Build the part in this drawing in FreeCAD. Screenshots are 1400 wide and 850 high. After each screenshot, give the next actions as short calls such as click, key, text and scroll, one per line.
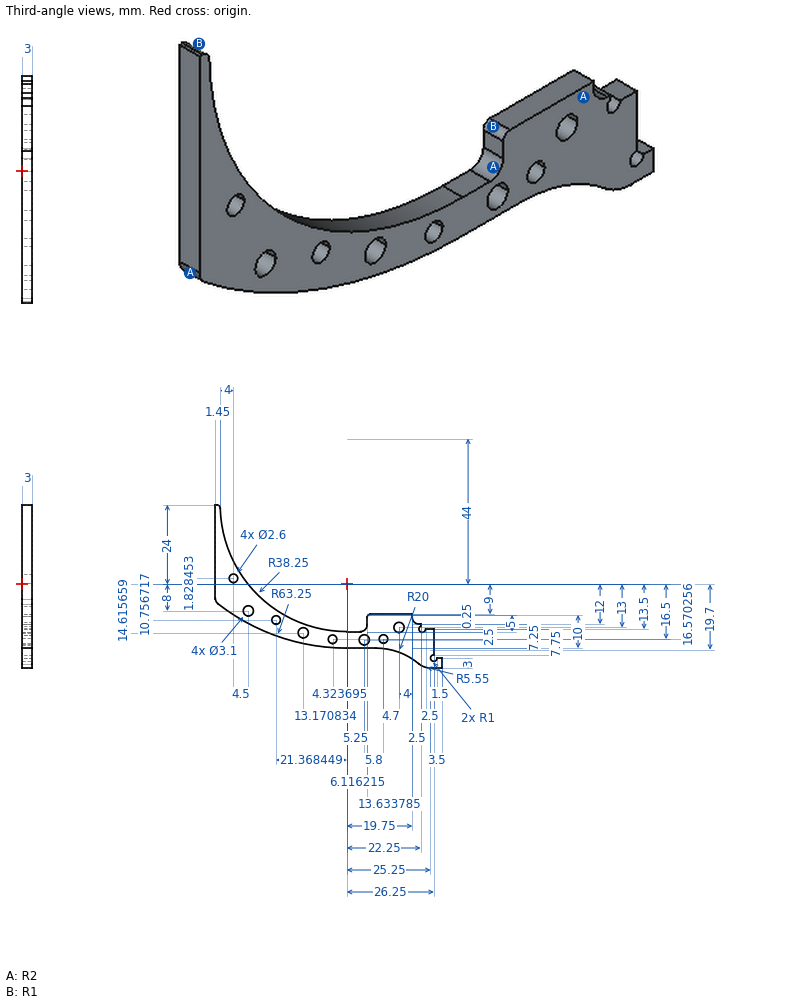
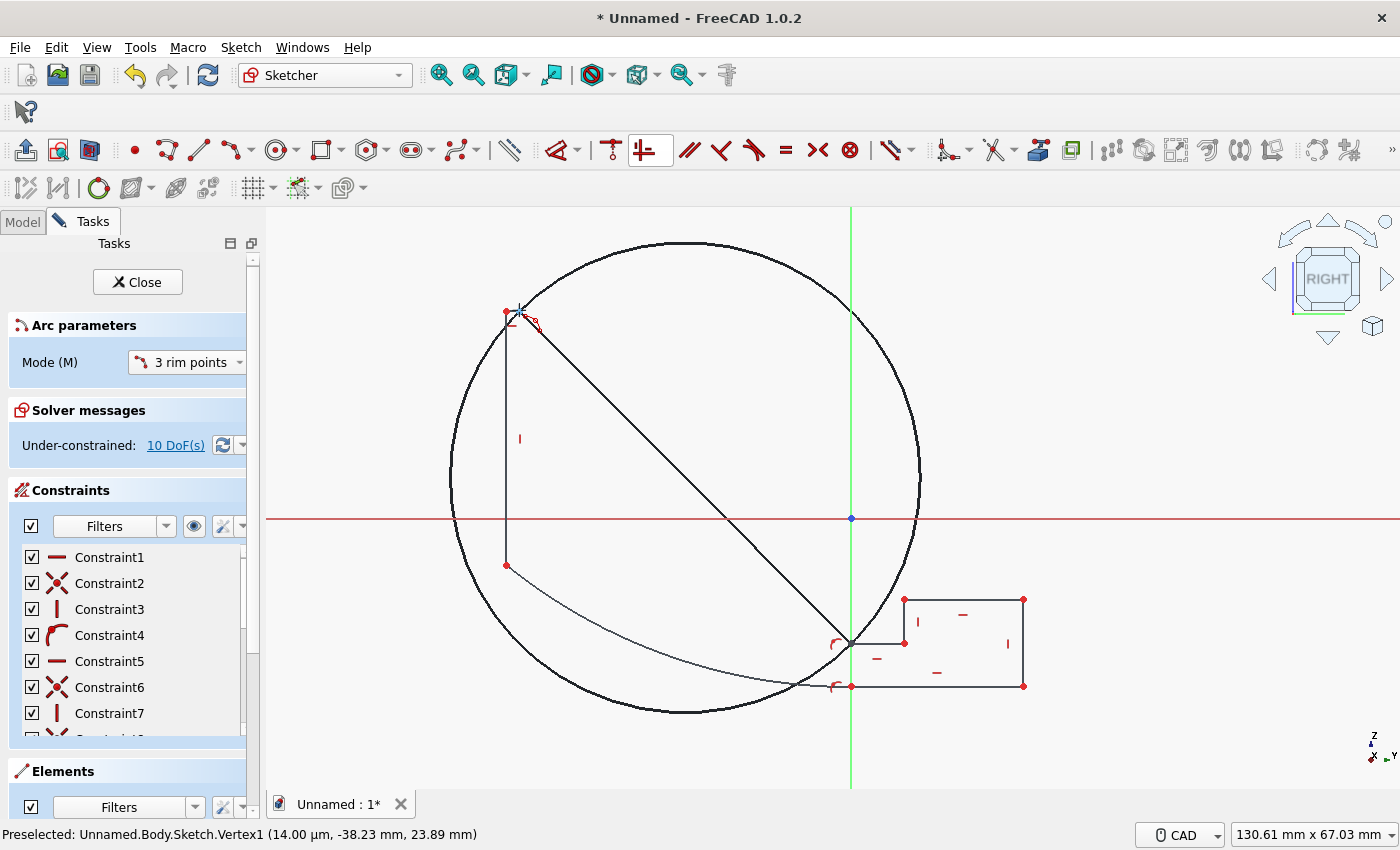
click(616, 545)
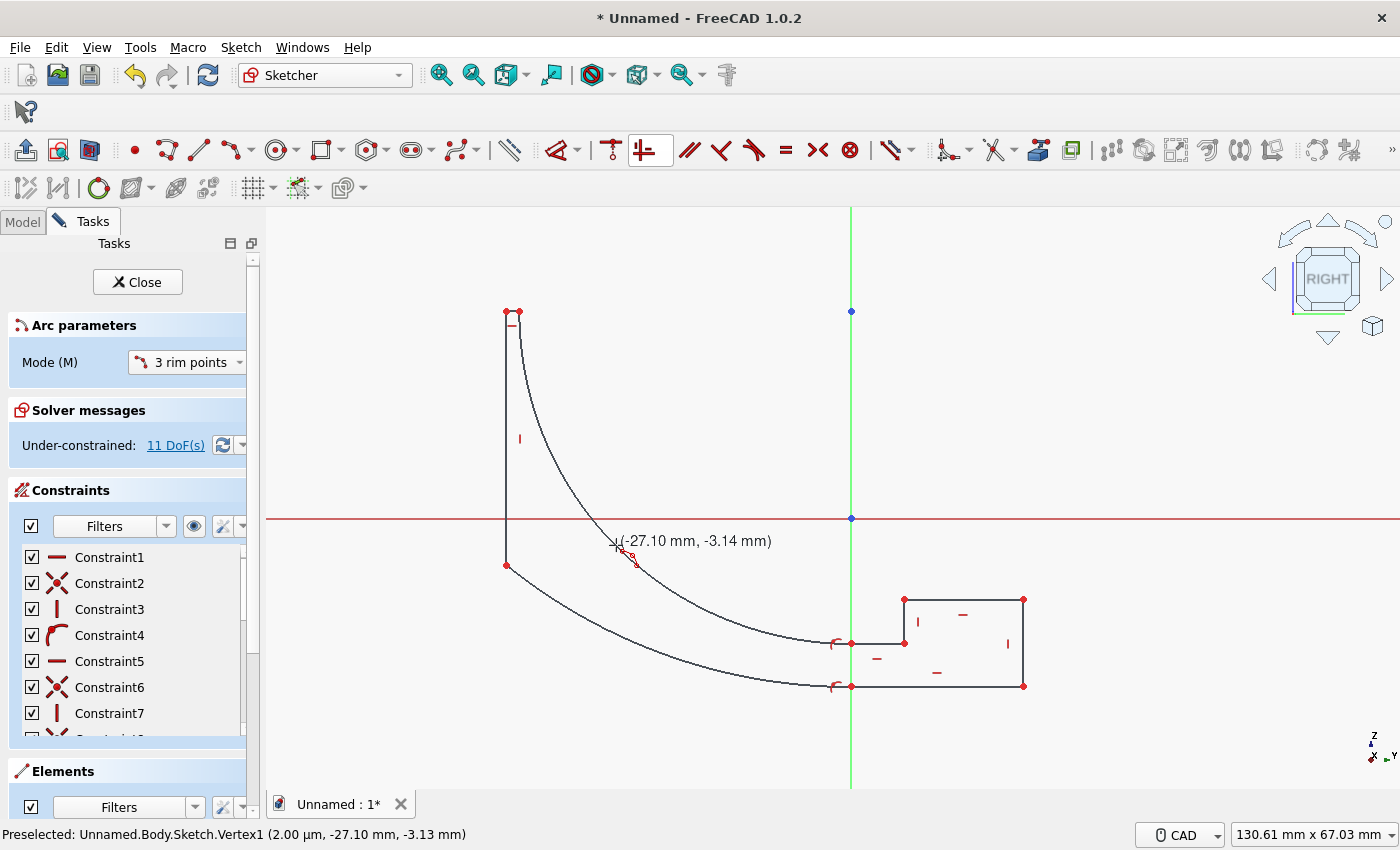
click(276, 150)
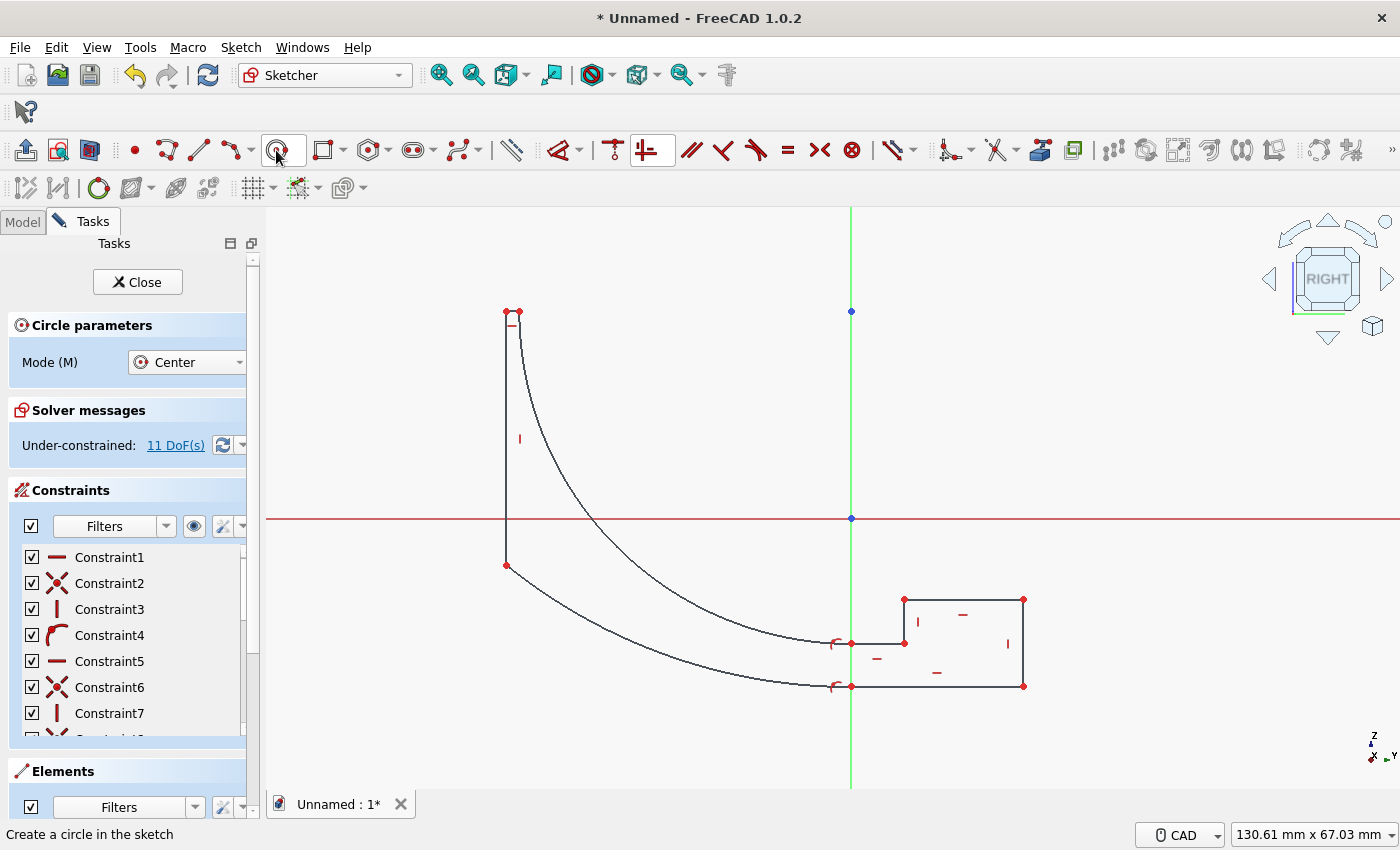
scroll(554, 503, up, 4)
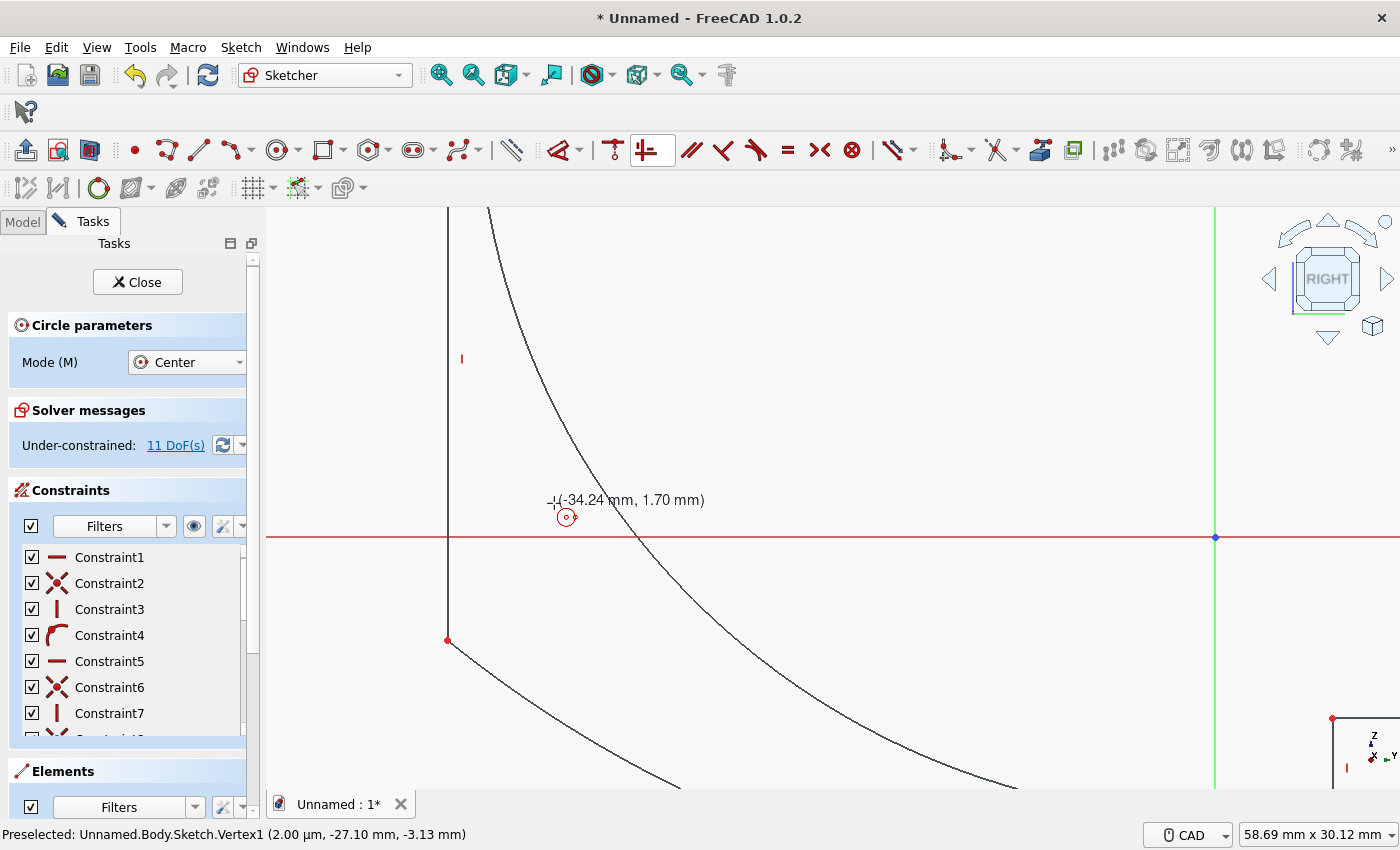
click(554, 502)
click(571, 484)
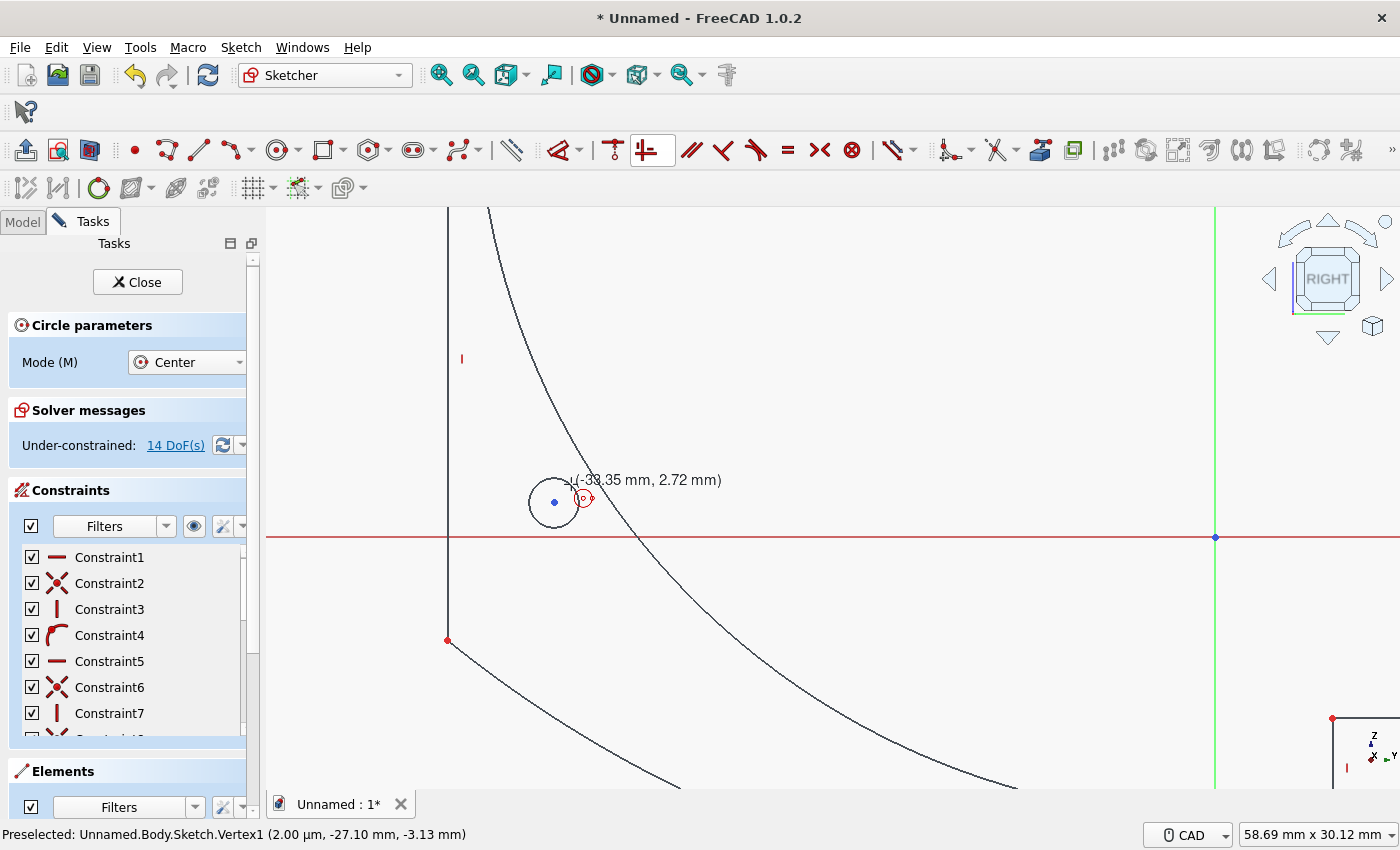
click(640, 692)
click(662, 671)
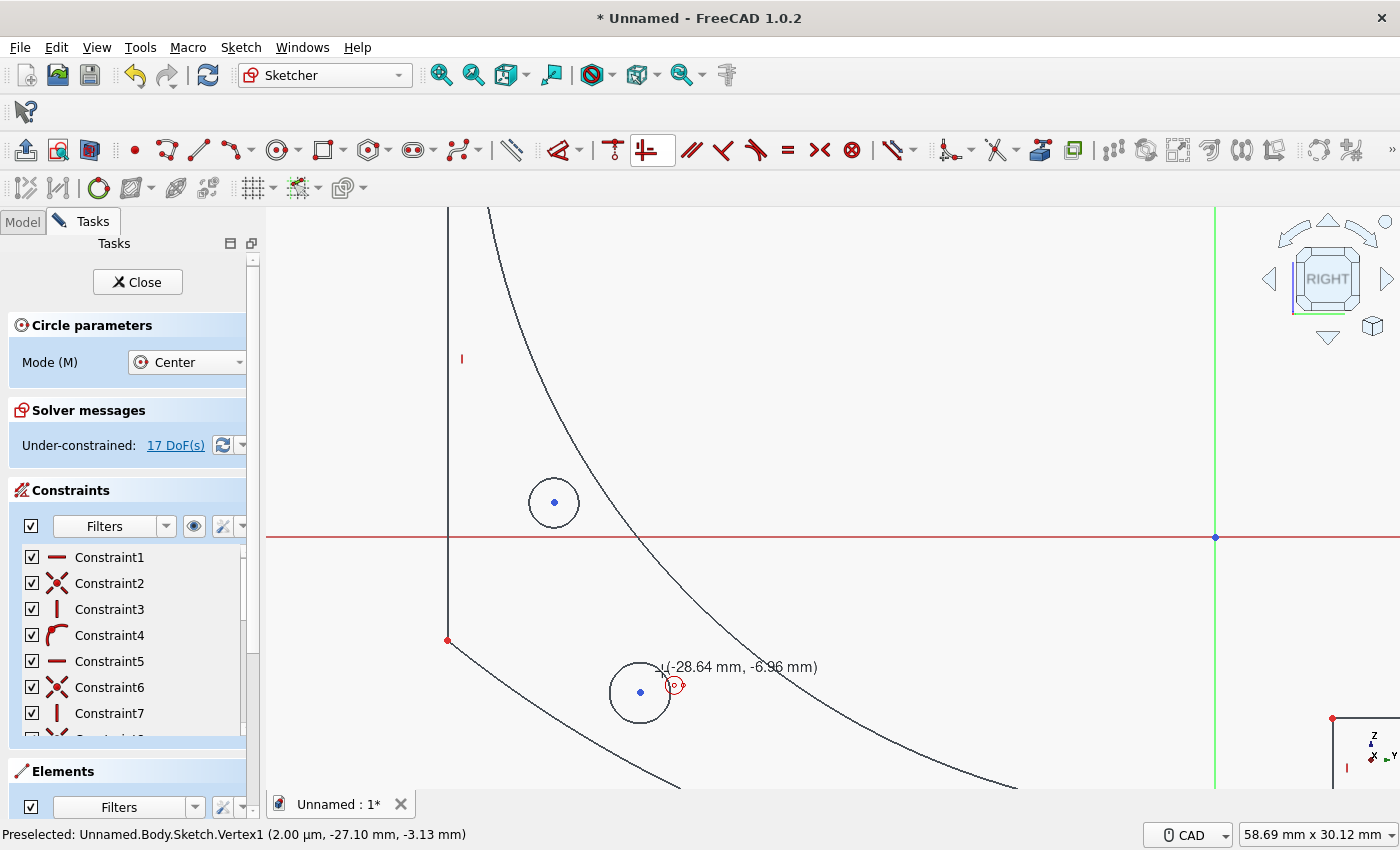
click(802, 745)
click(820, 728)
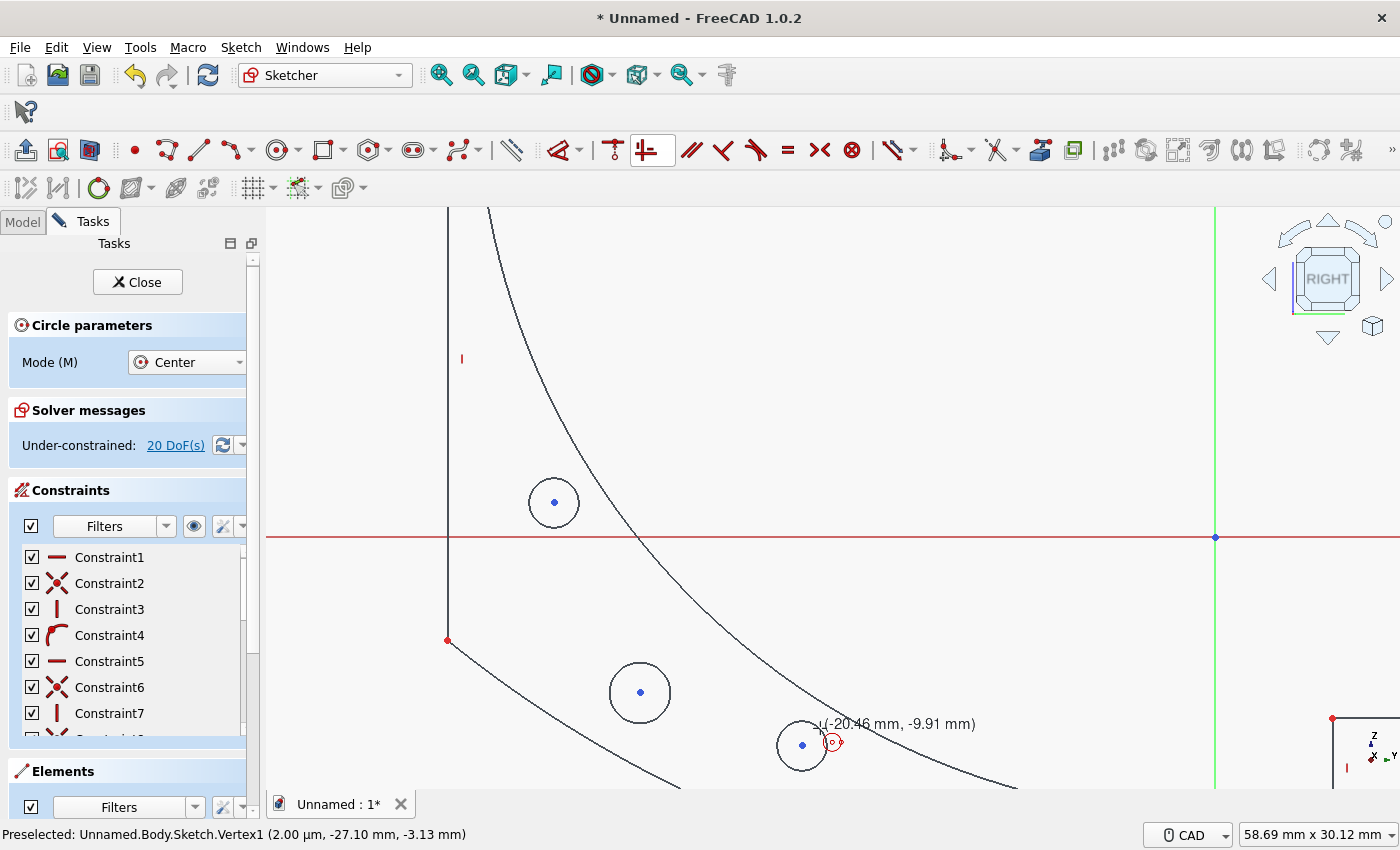
scroll(554, 503, down, 4)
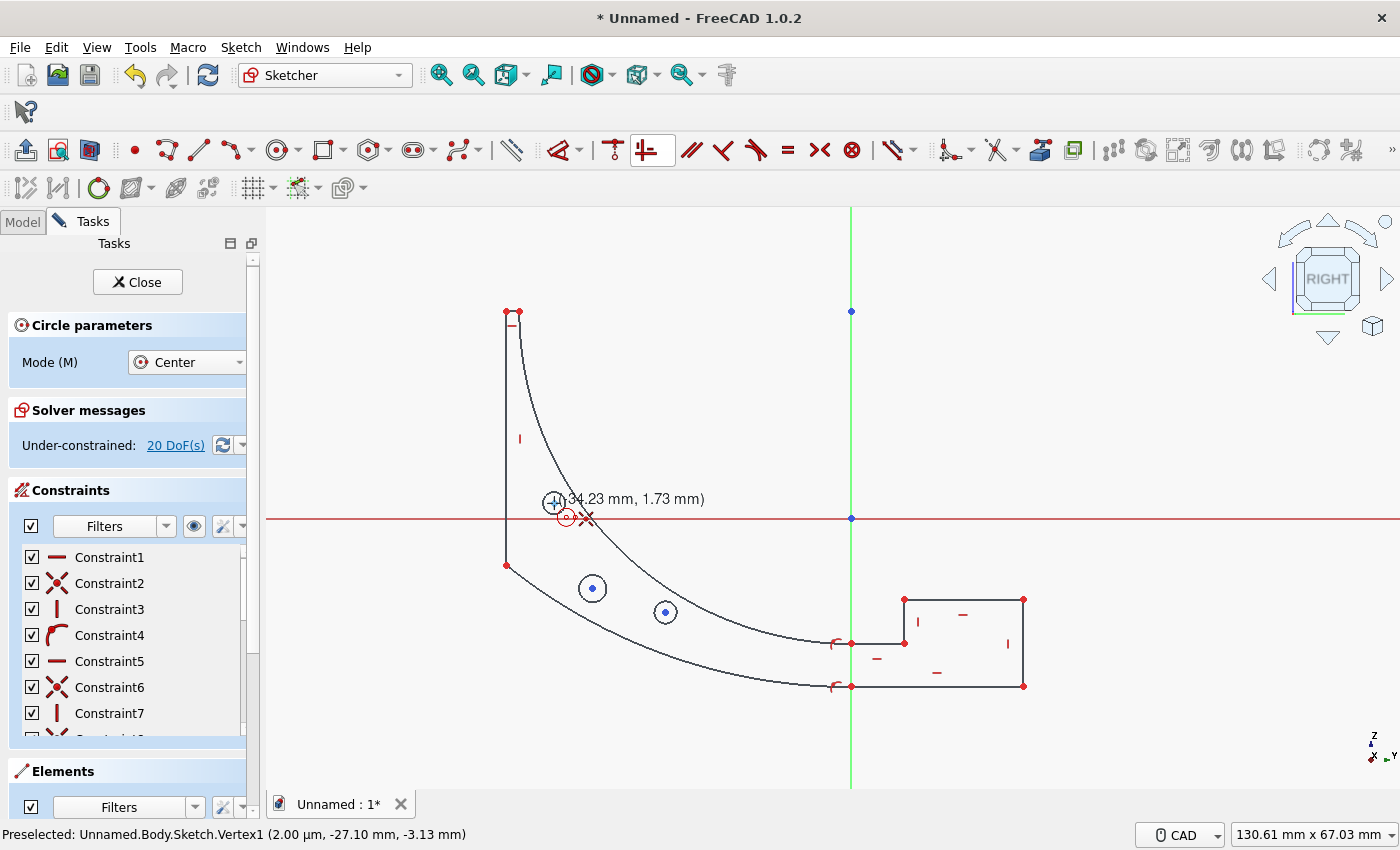
scroll(737, 646, up, 3)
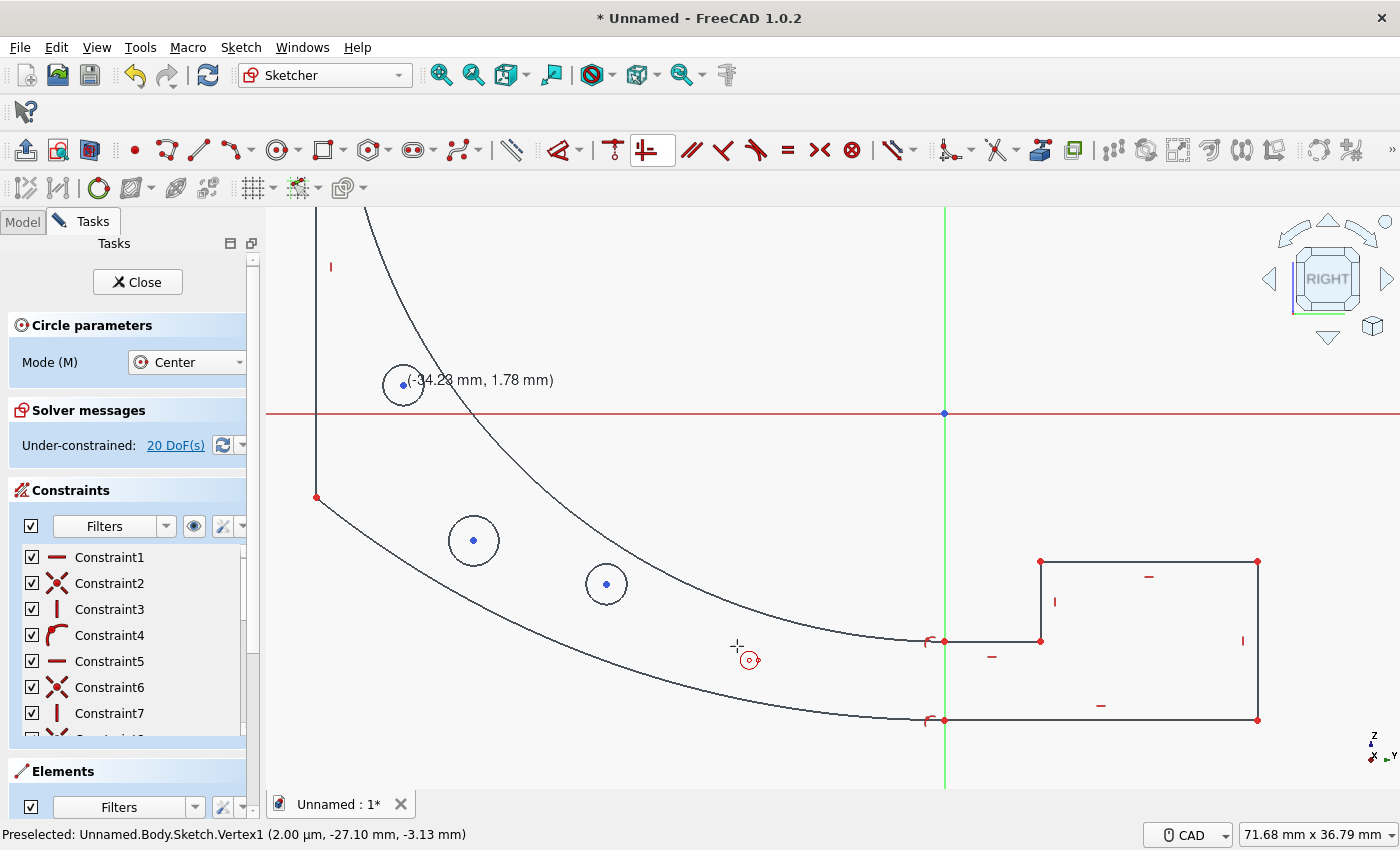
click(737, 645)
click(754, 627)